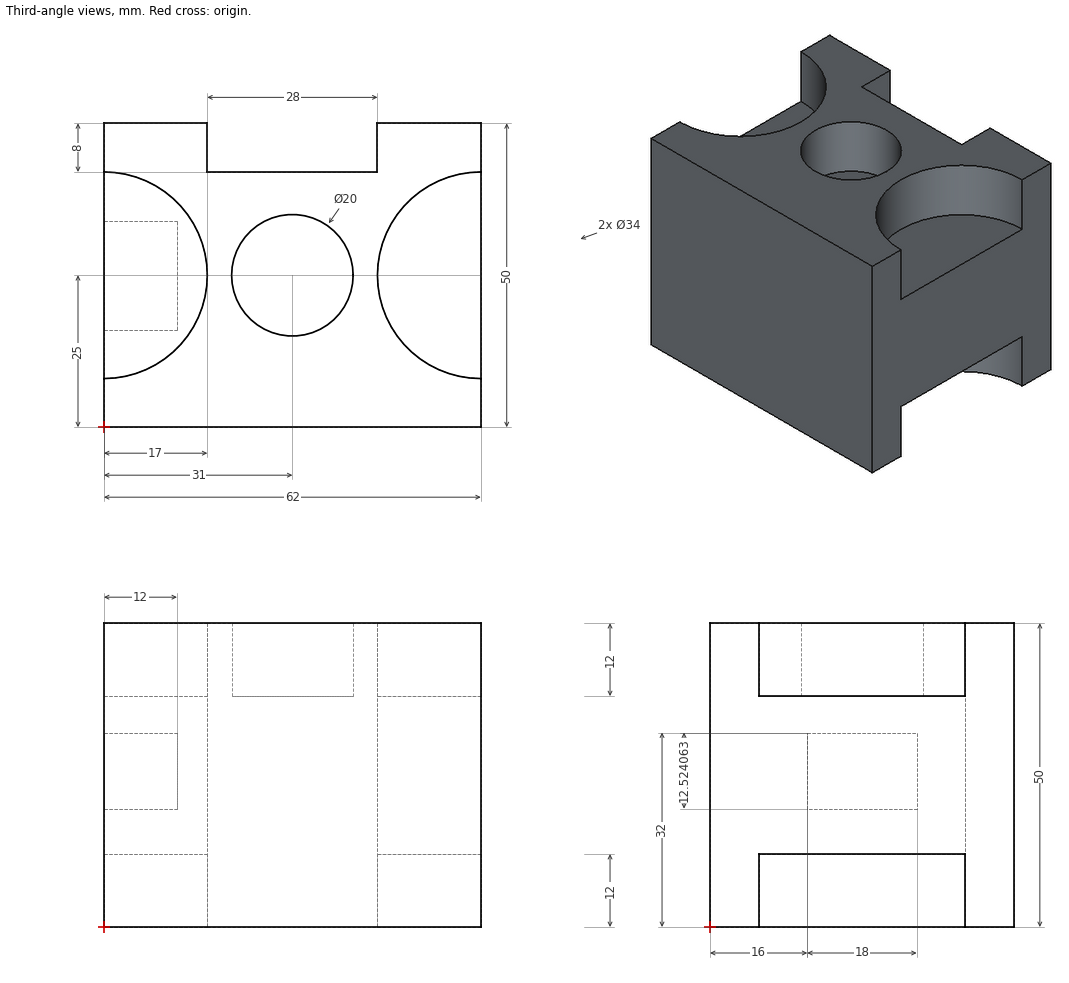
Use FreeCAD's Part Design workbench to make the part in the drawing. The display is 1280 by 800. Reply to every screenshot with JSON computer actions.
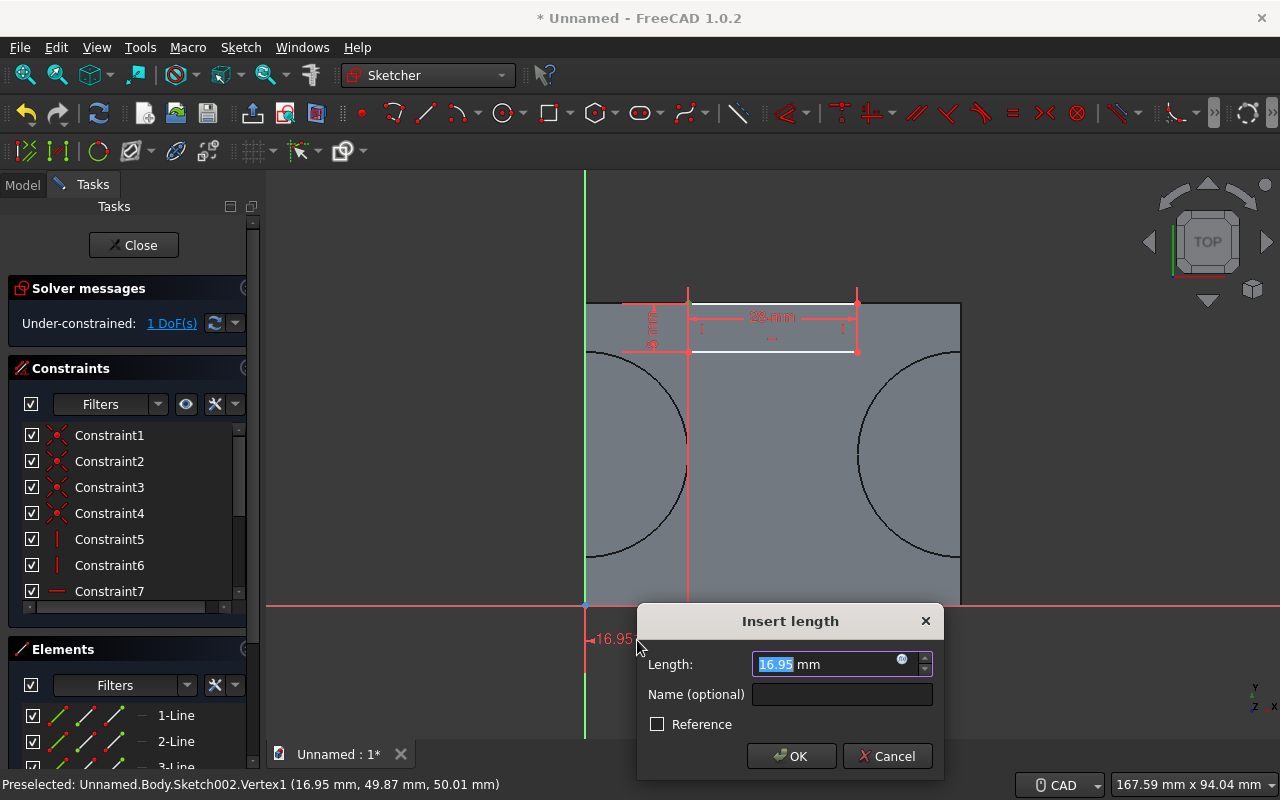
{"action": "type", "text": "17"}
{"action": "key", "text": "Return"}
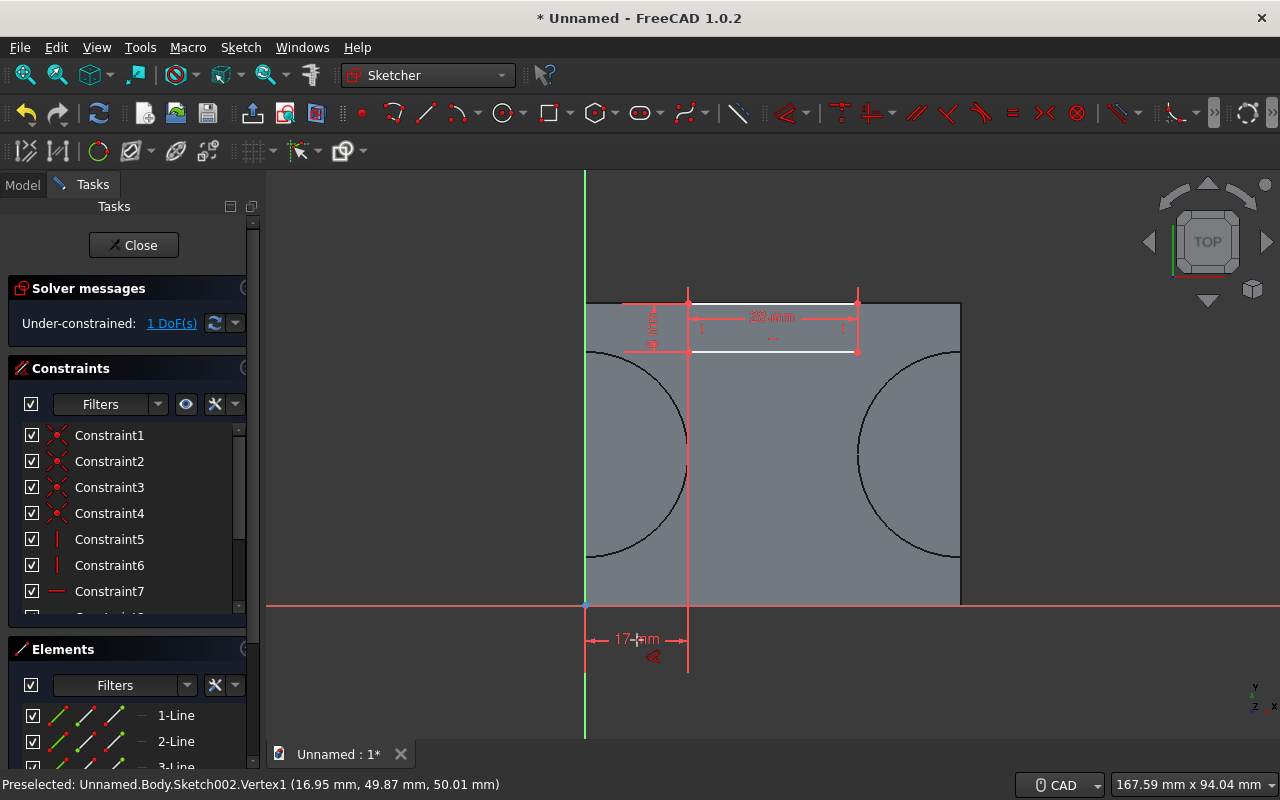
{"action": "left_click", "coordinate": [688, 304]}
{"action": "left_click", "coordinate": [551, 455]}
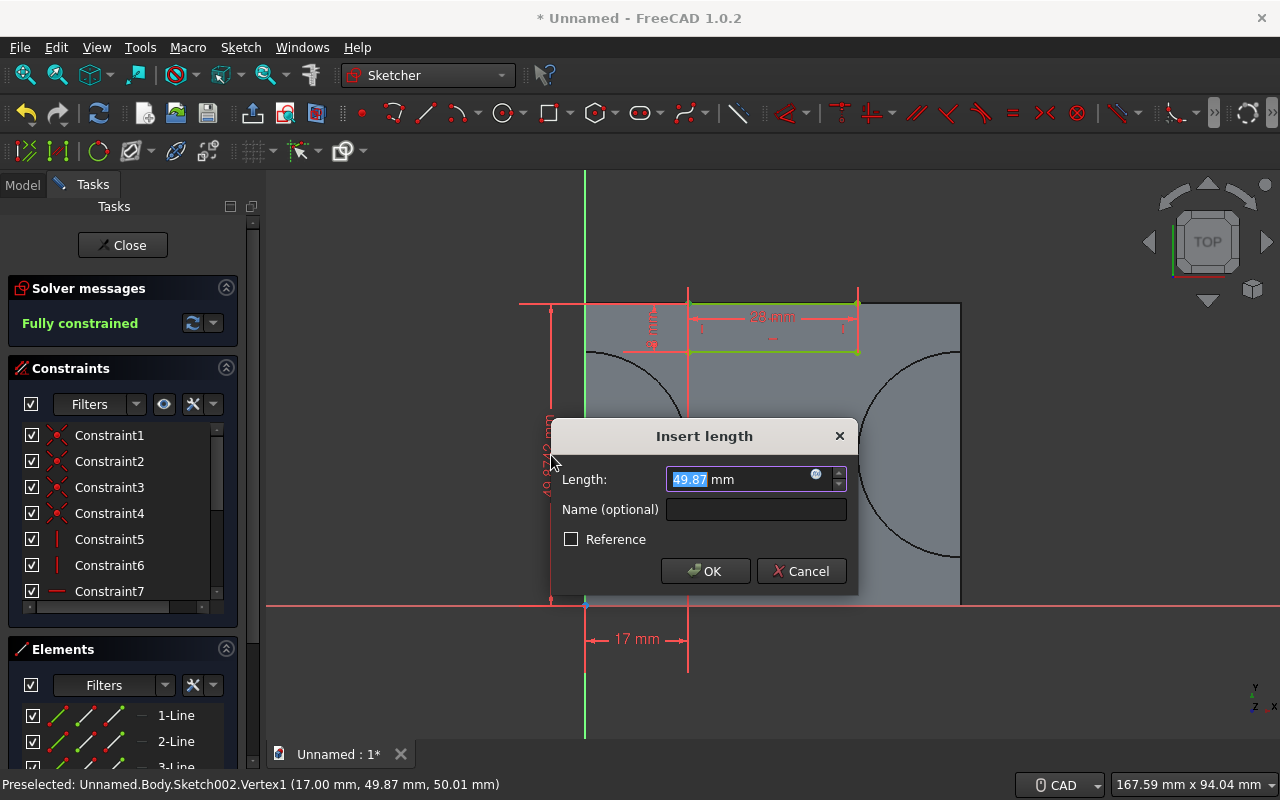
{"action": "type", "text": "50"}
{"action": "key", "text": "Return"}
{"action": "key", "text": "Escape"}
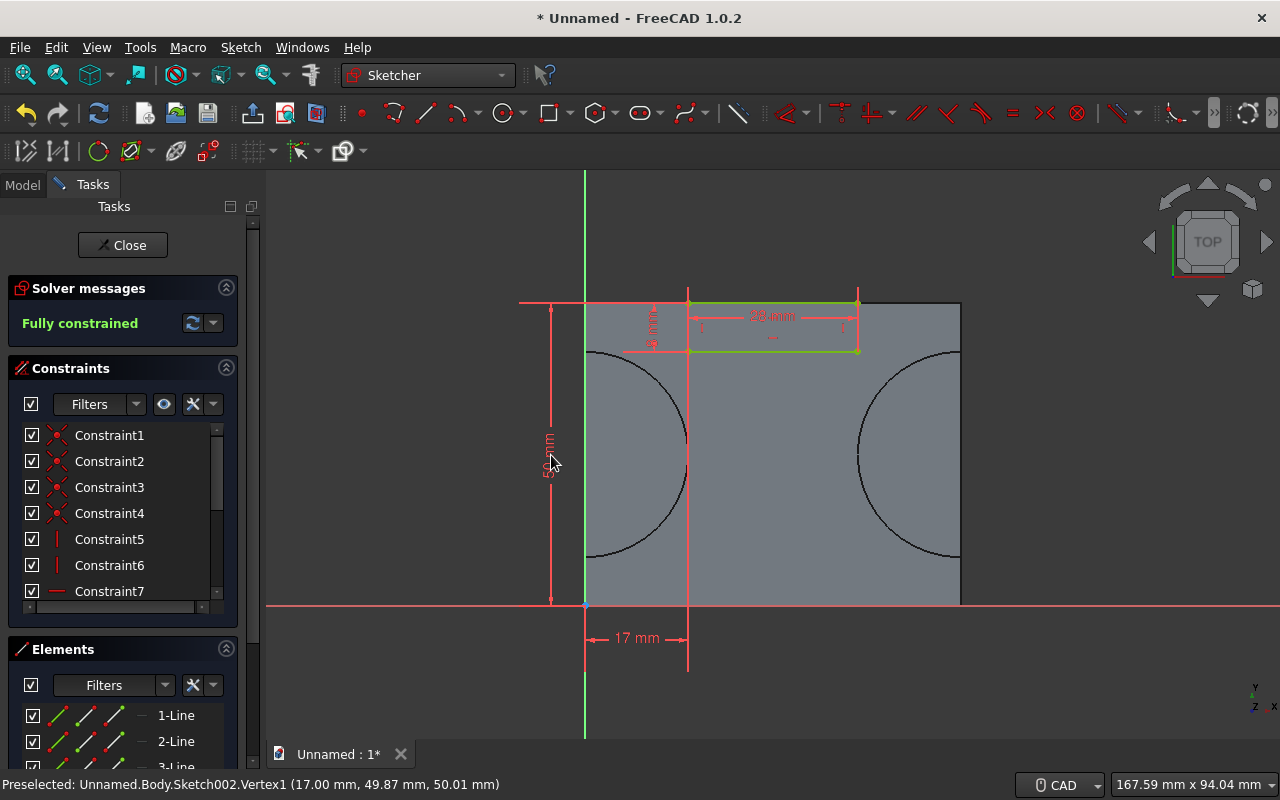
{"action": "left_click", "coordinate": [123, 245]}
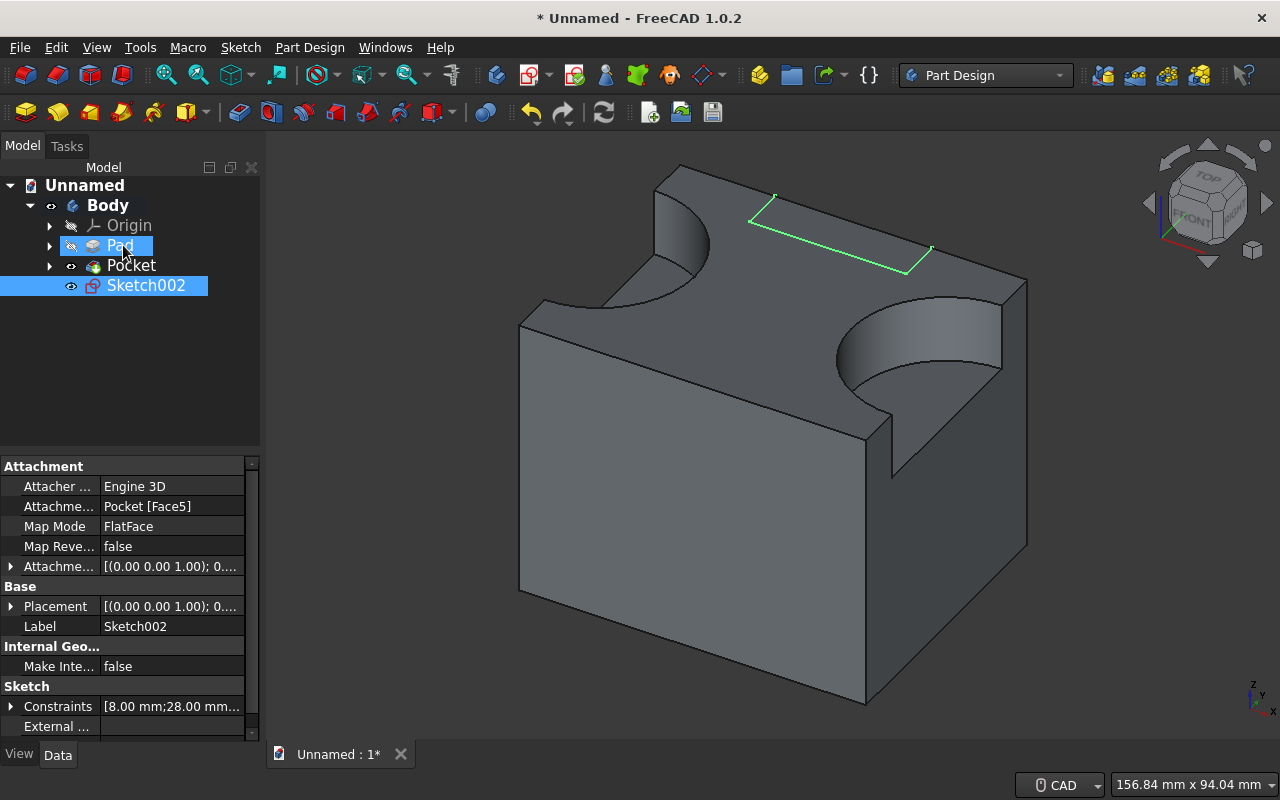
{"action": "left_click", "coordinate": [240, 112]}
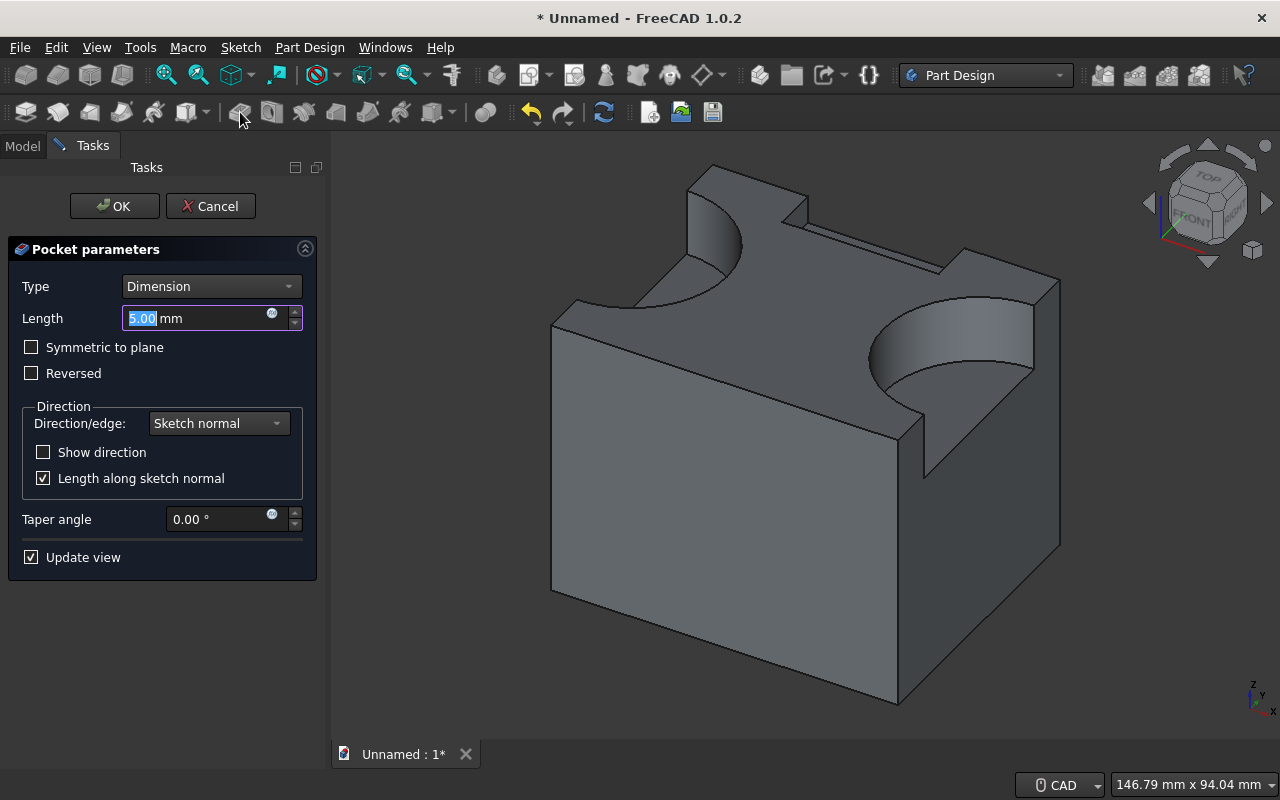
{"action": "left_click", "coordinate": [212, 286]}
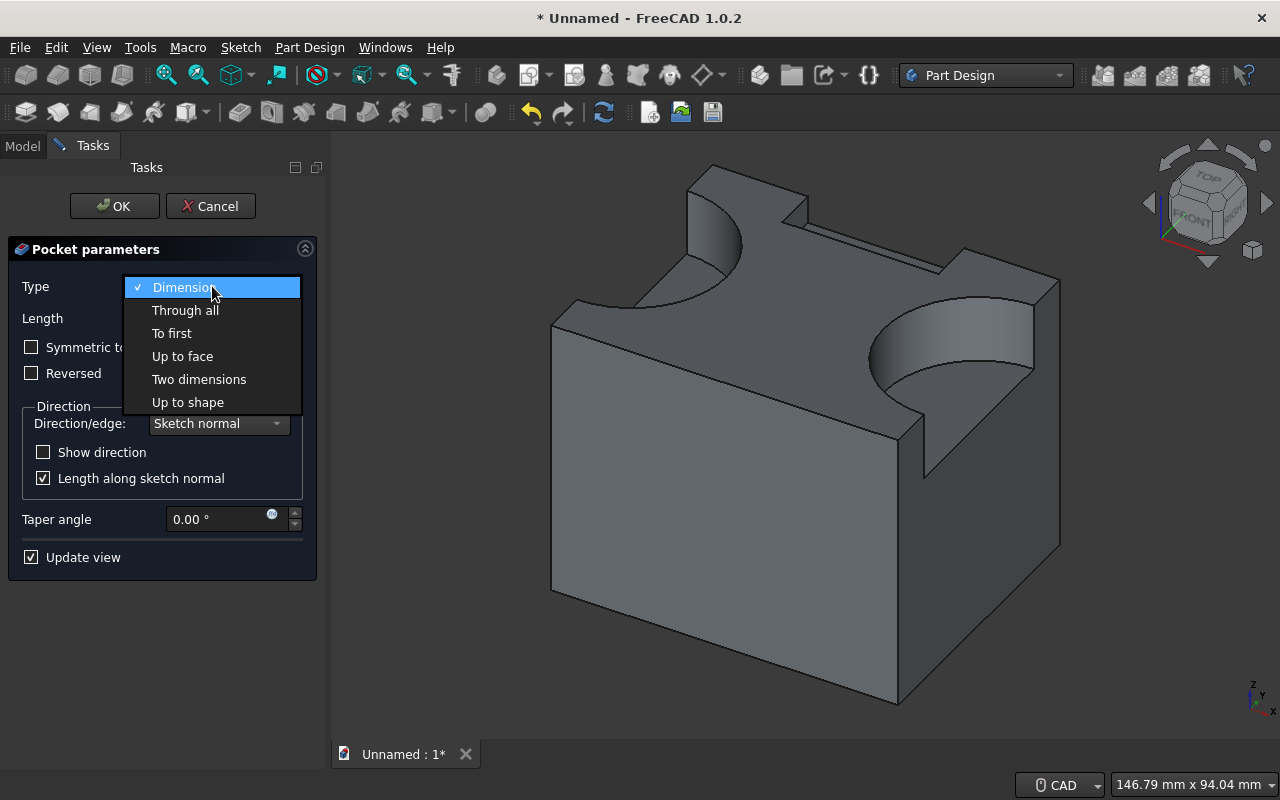
{"action": "left_click", "coordinate": [212, 310]}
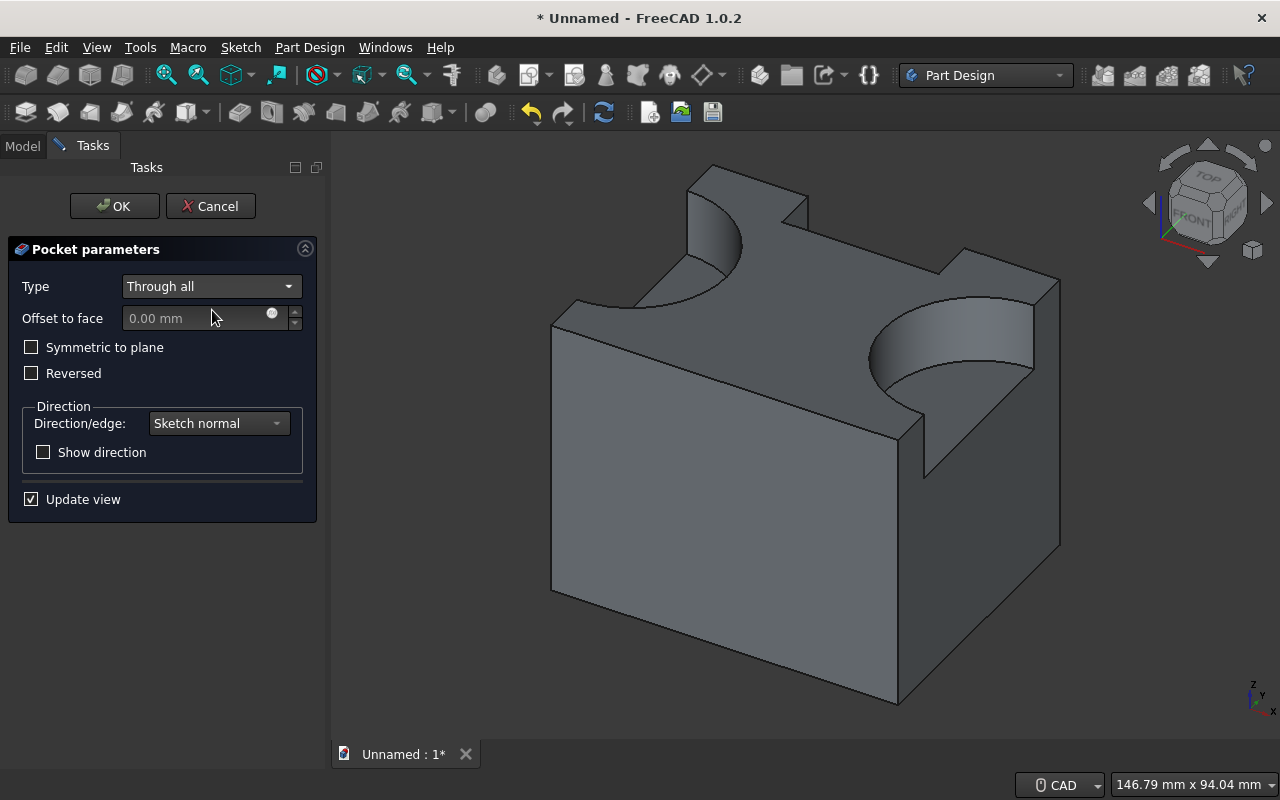
{"action": "left_click", "coordinate": [115, 206]}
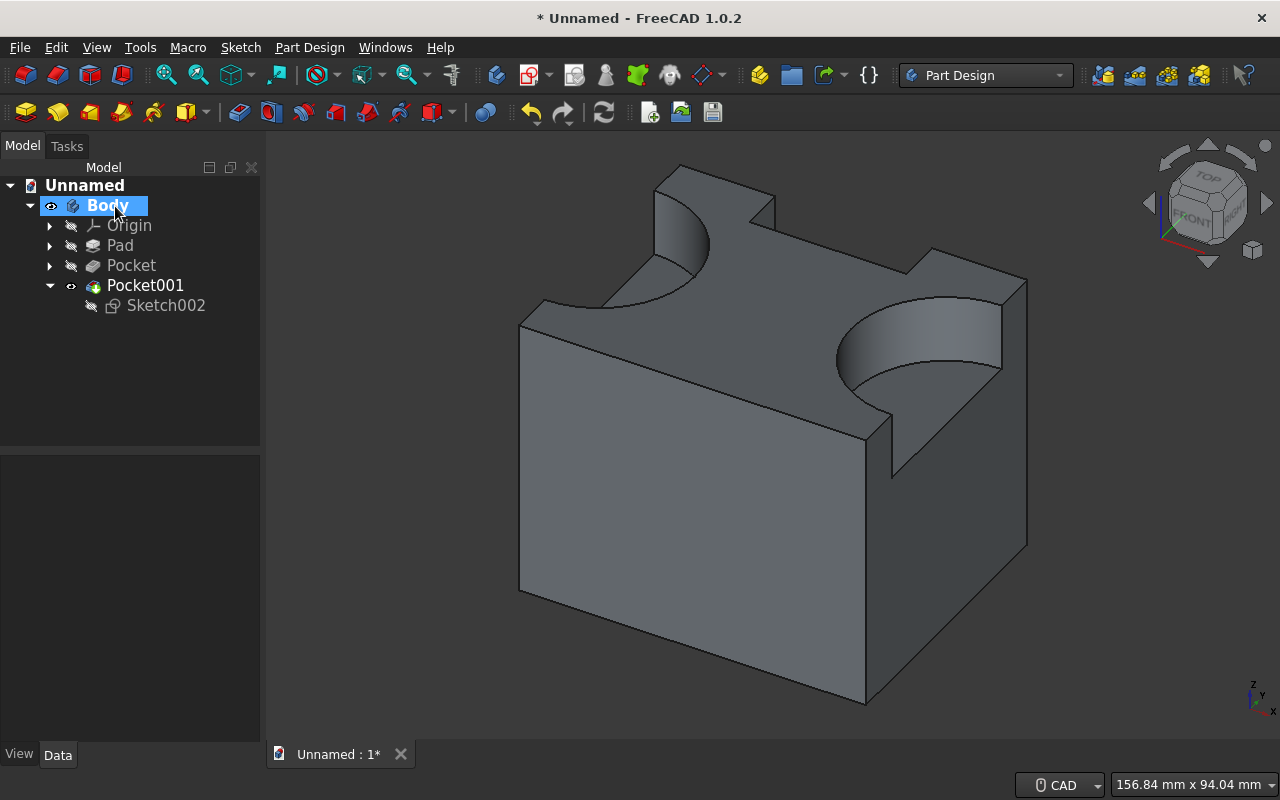
{"action": "left_click", "coordinate": [530, 76]}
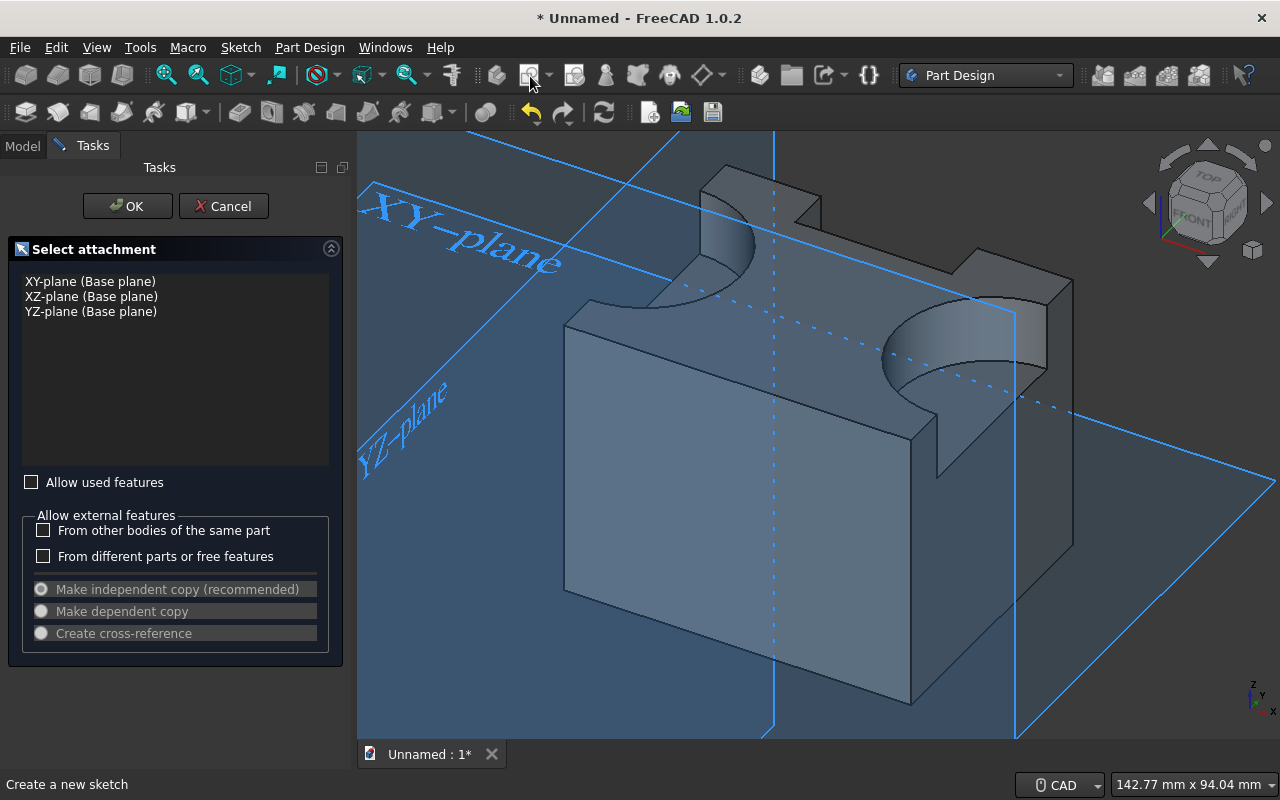
{"action": "left_click", "coordinate": [82, 312]}